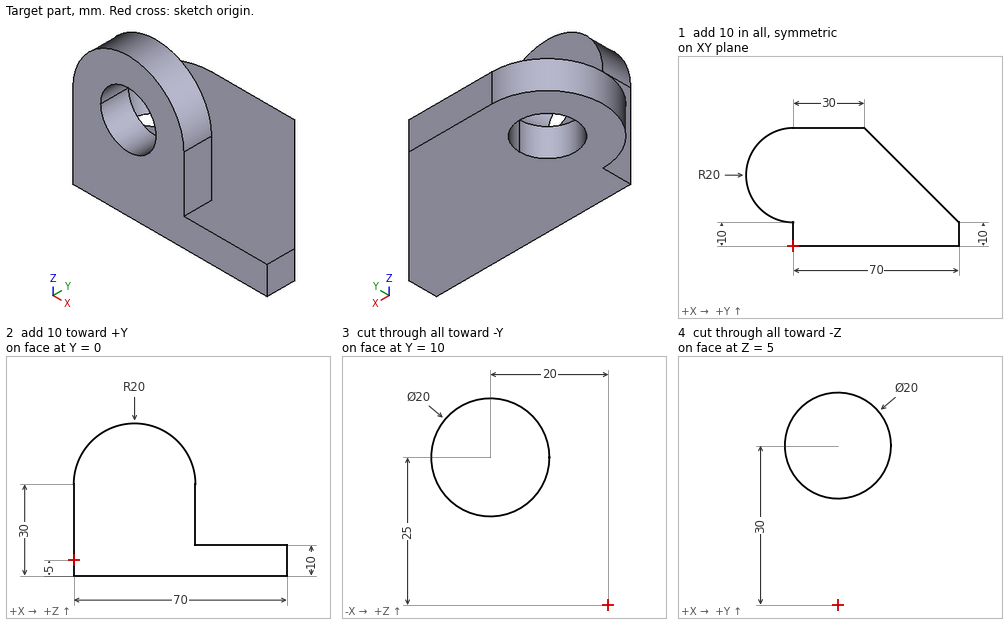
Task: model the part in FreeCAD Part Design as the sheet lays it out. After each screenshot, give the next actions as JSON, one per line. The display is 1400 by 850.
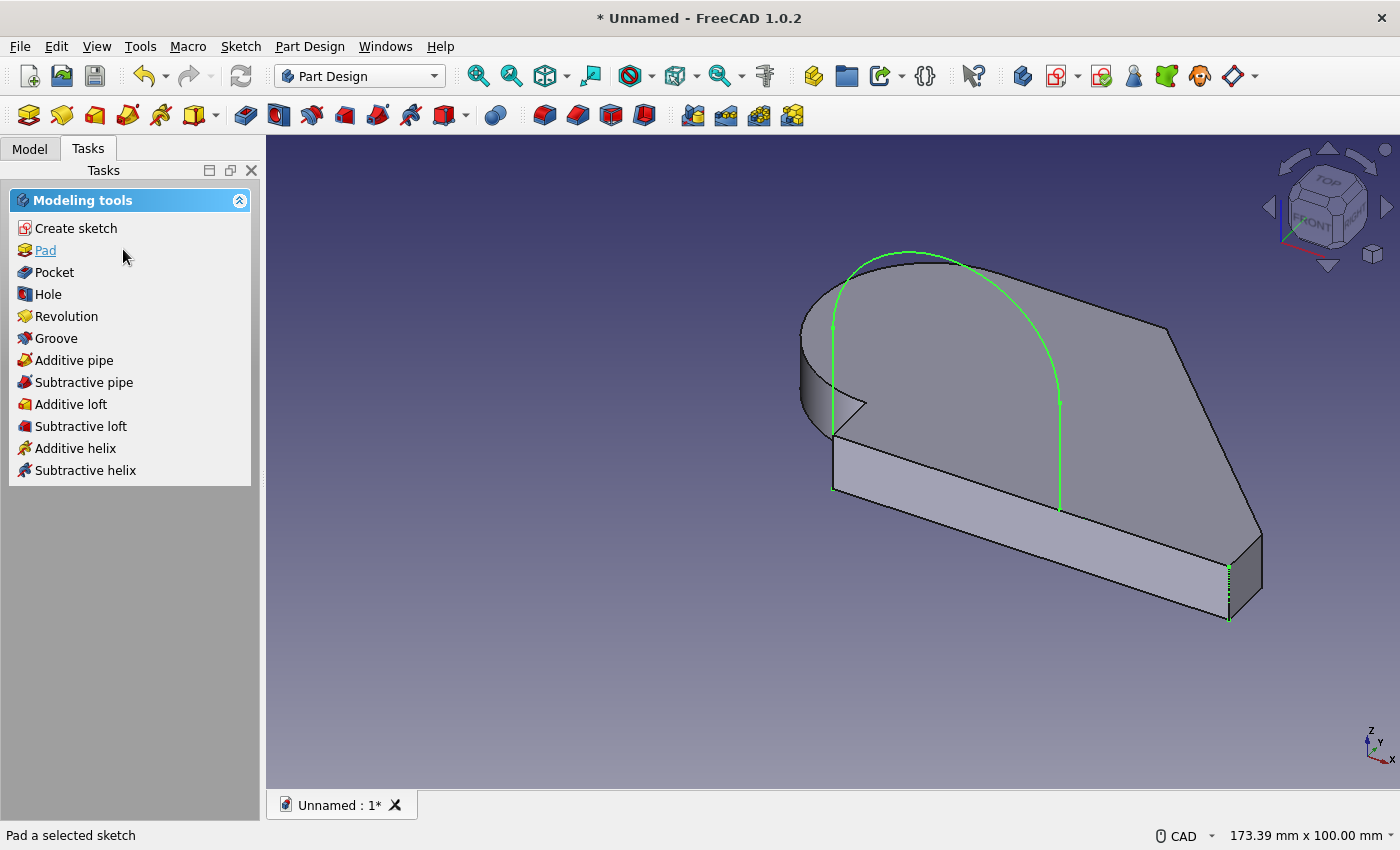
{"action": "left_click", "coordinate": [29, 116]}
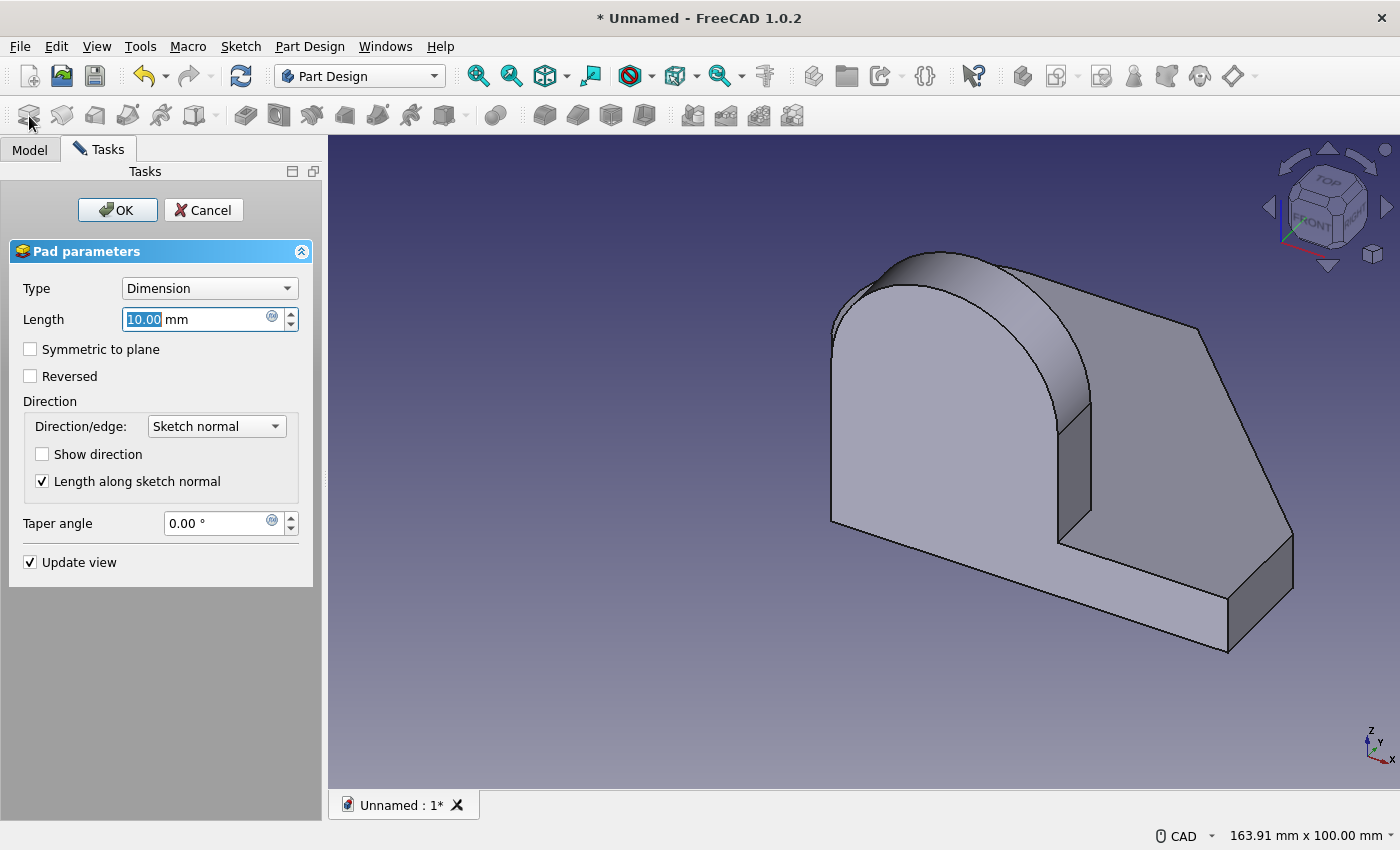
{"action": "type", "text": "10"}
{"action": "key", "text": "Tab"}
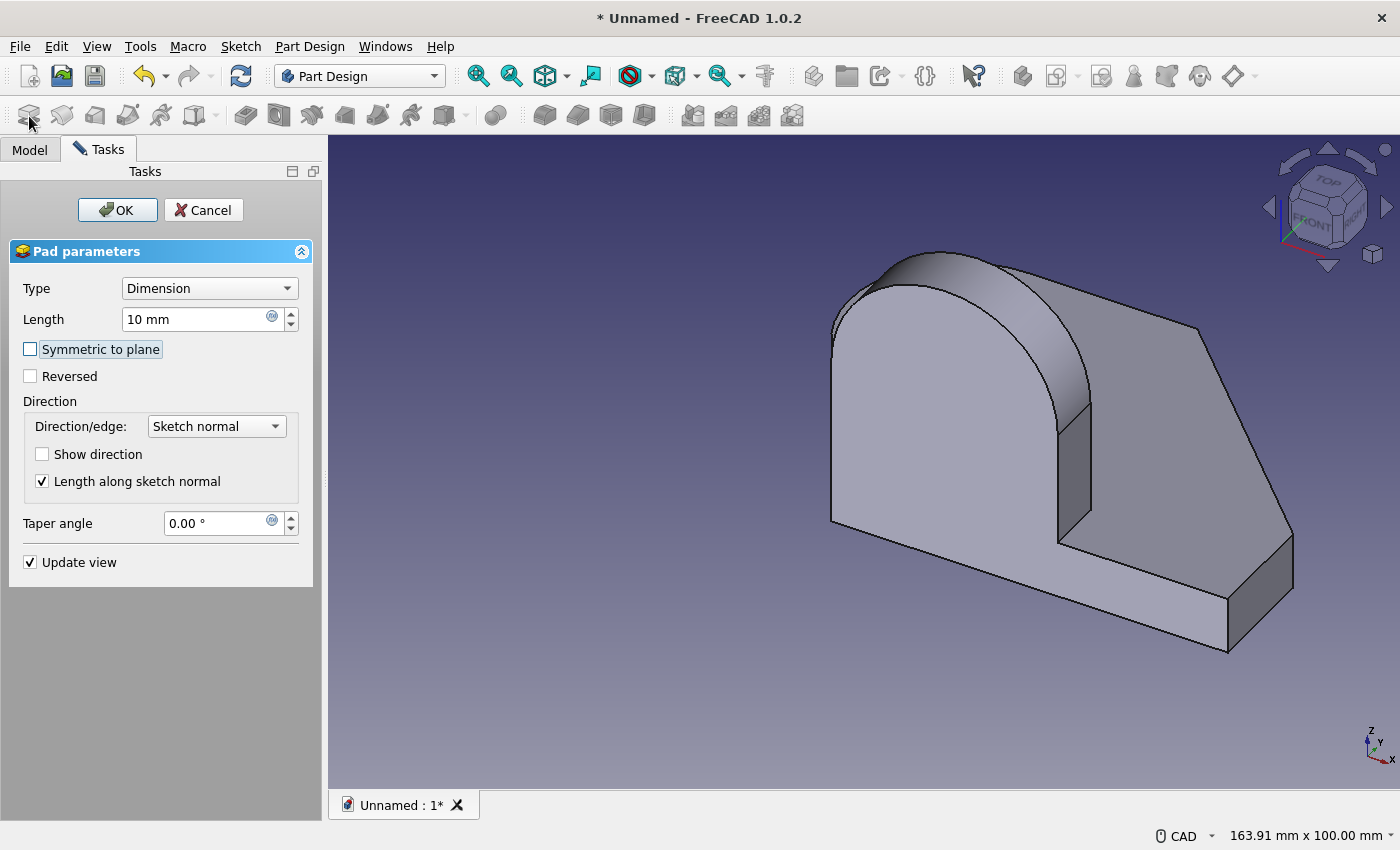
{"action": "left_click", "coordinate": [31, 376]}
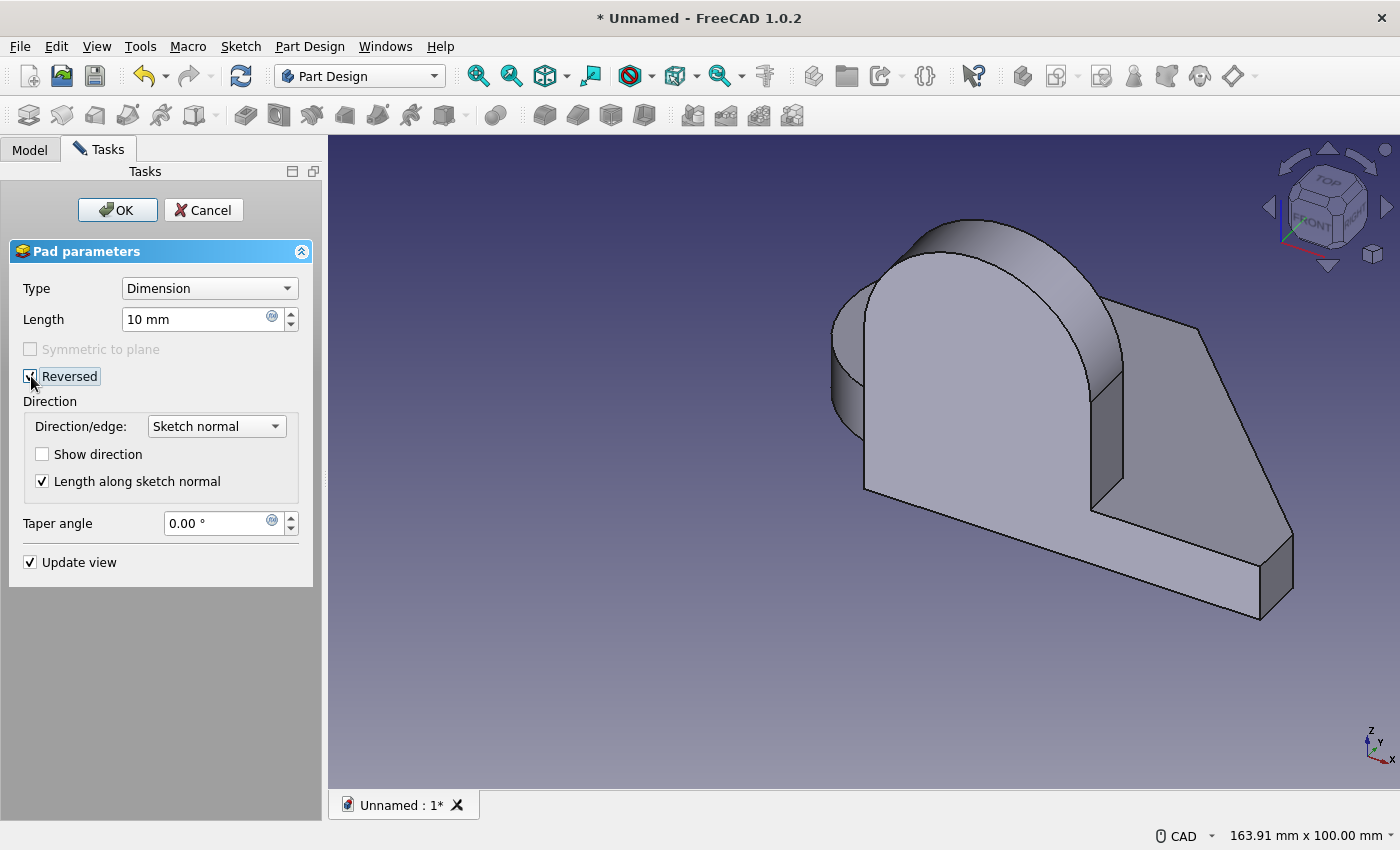
{"action": "left_click", "coordinate": [118, 210]}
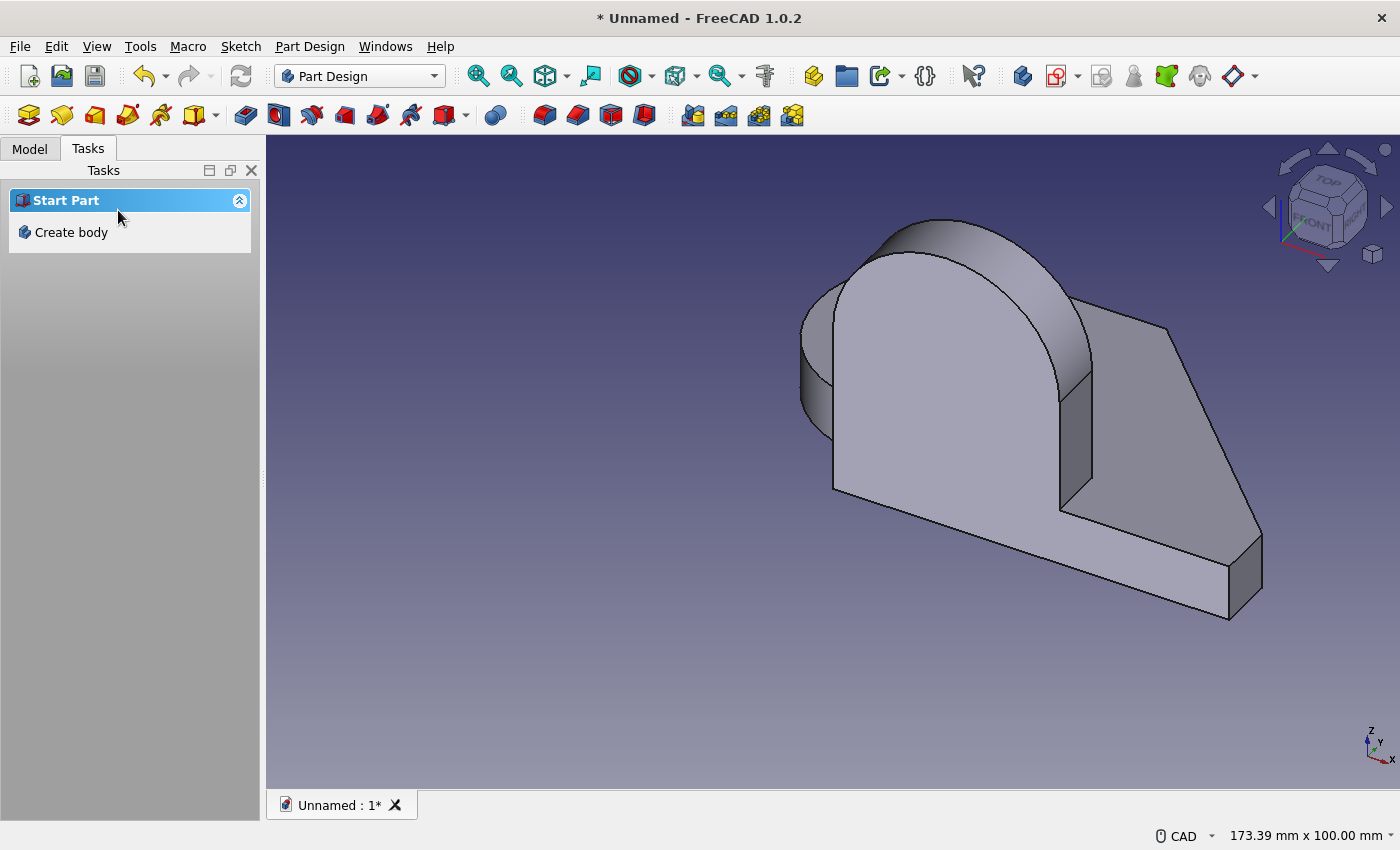
{"action": "left_click", "coordinate": [479, 76]}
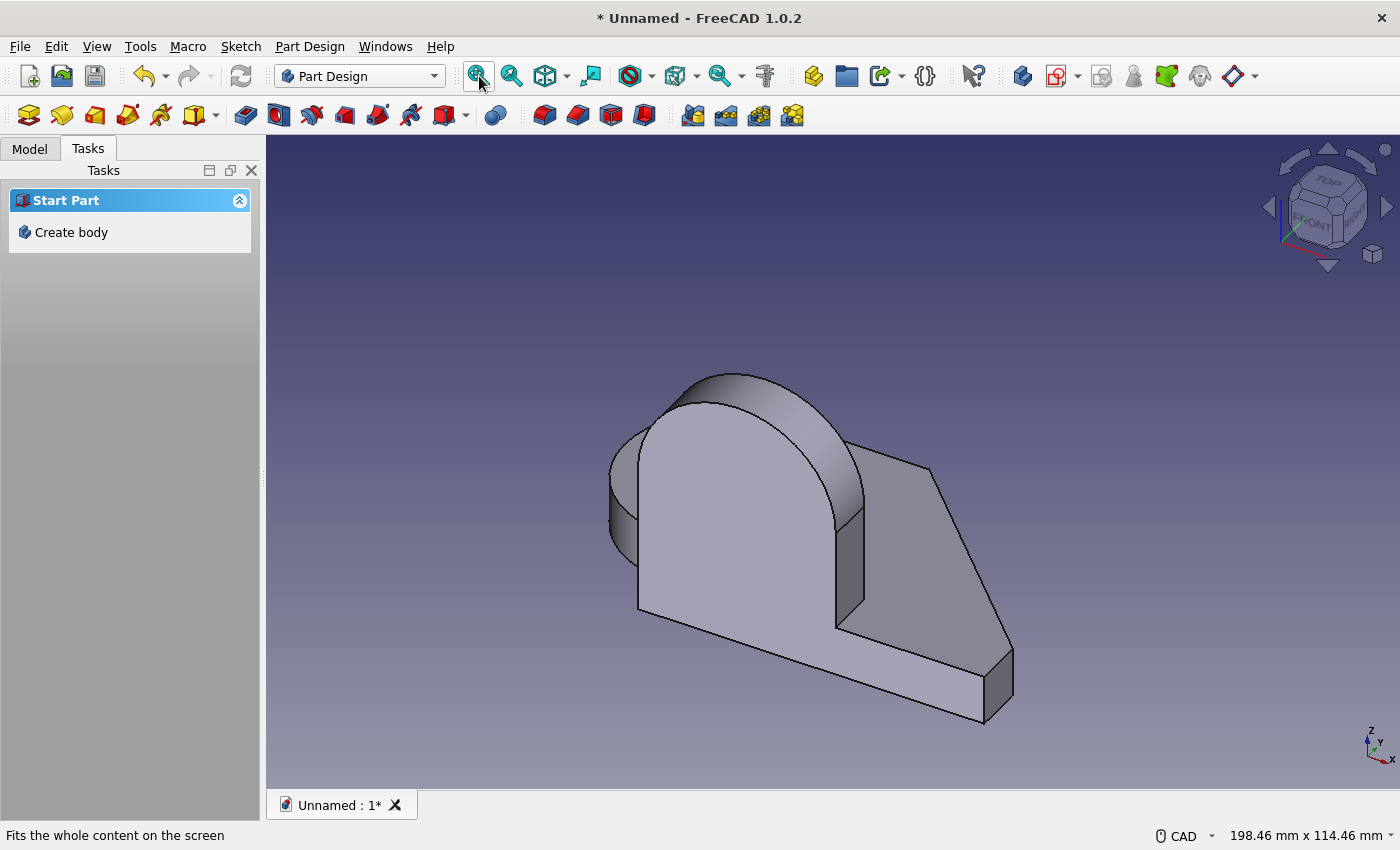
{"action": "key", "text": "4"}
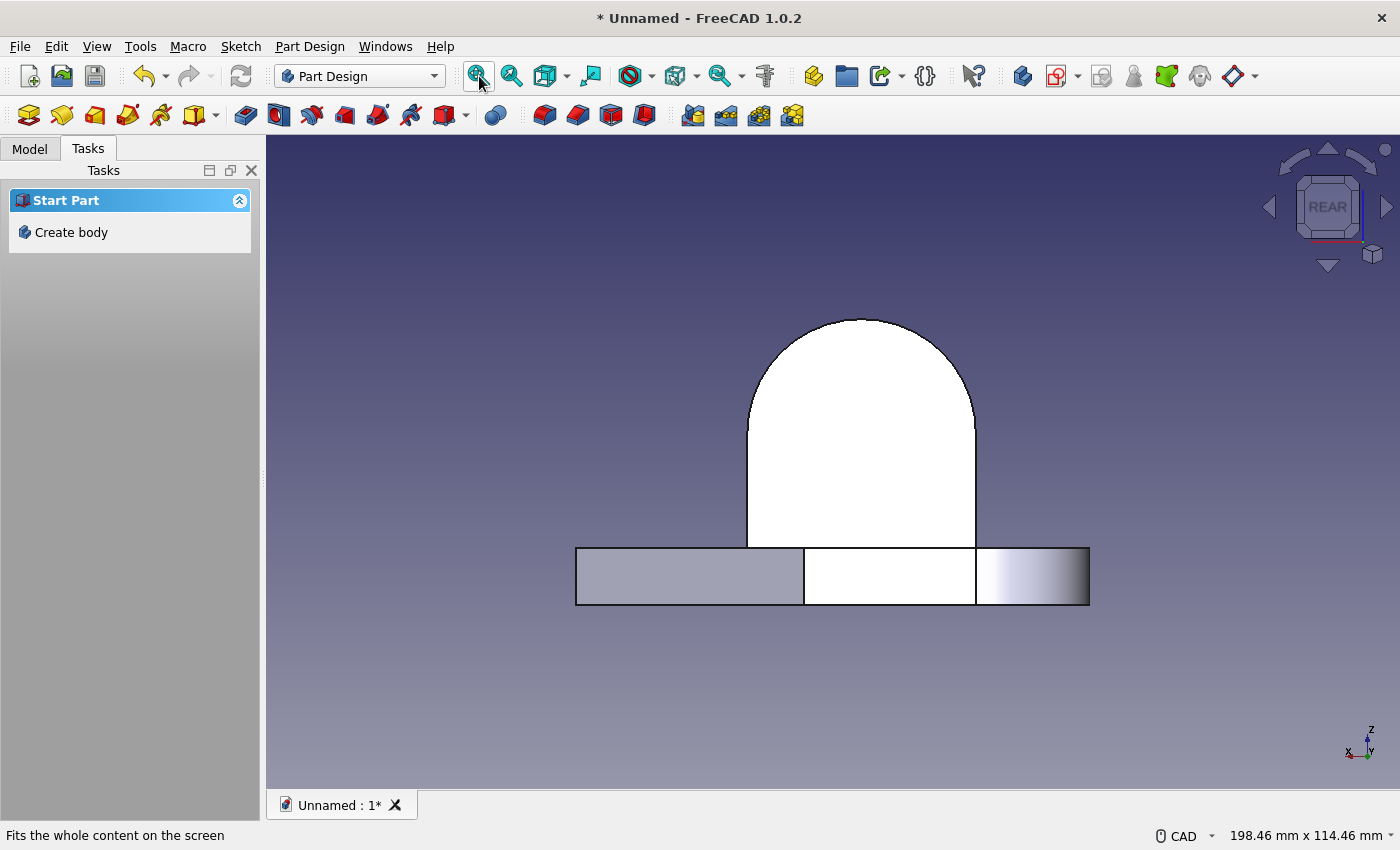
{"action": "left_click", "coordinate": [862, 432]}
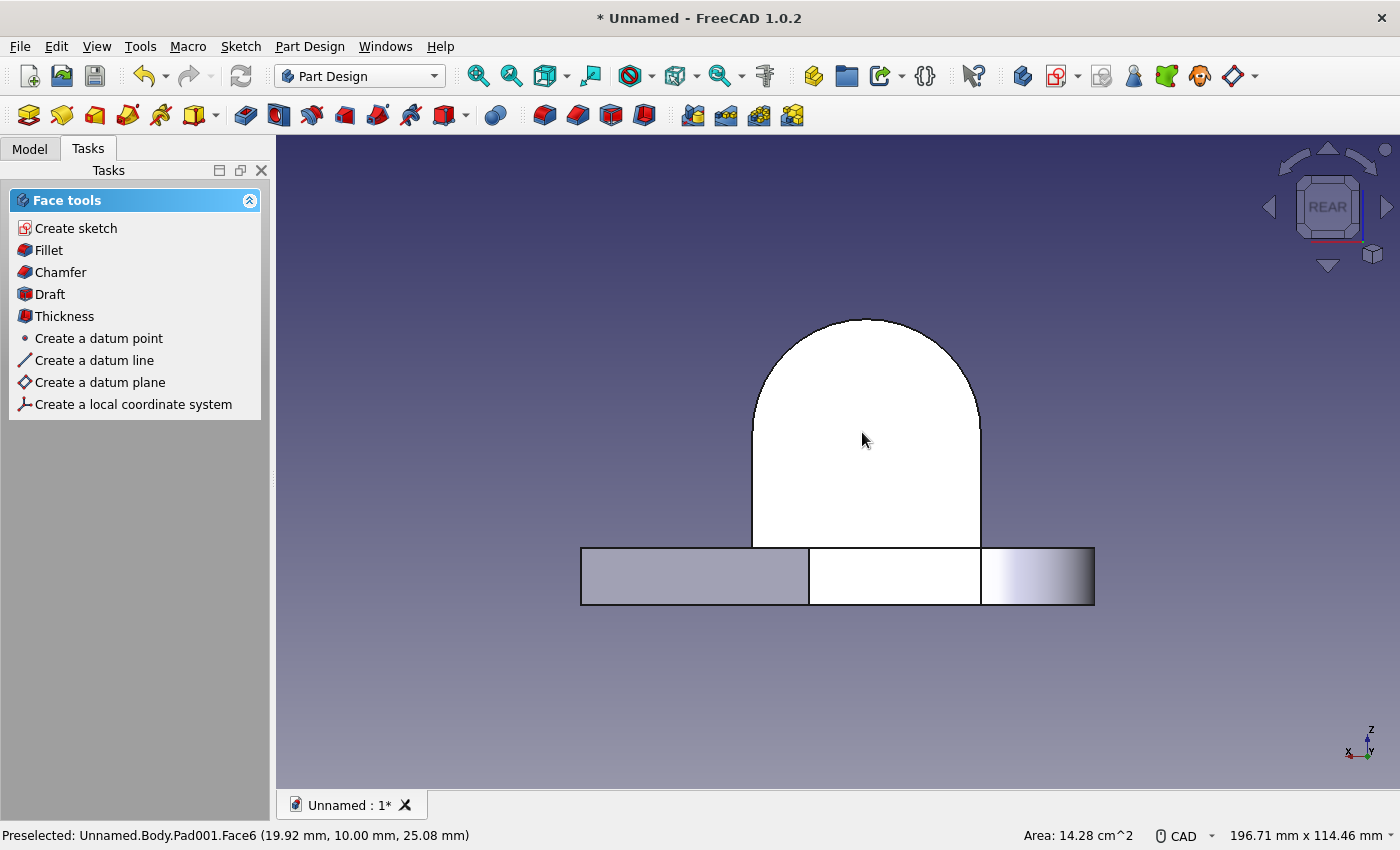
{"action": "left_click", "coordinate": [1056, 76]}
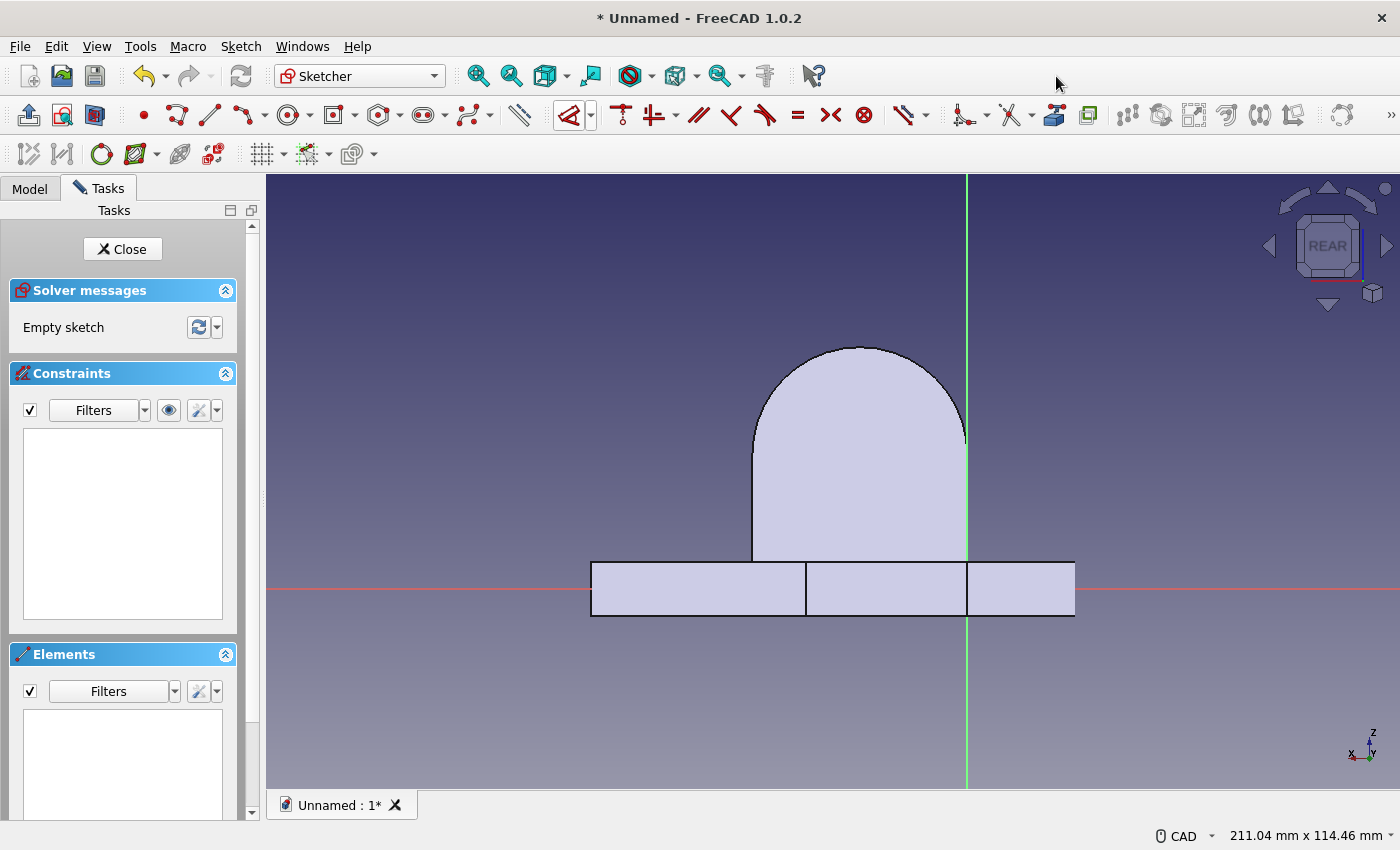
{"action": "scroll", "coordinate": [986, 506], "scroll_direction": "up", "scroll_amount": 4}